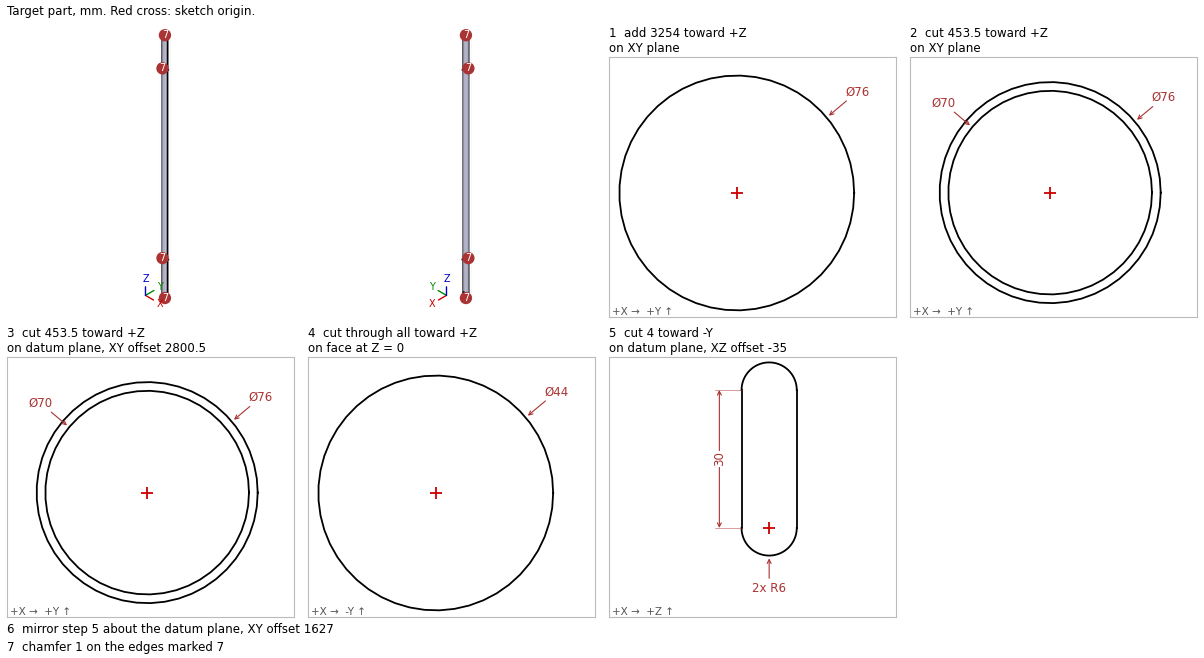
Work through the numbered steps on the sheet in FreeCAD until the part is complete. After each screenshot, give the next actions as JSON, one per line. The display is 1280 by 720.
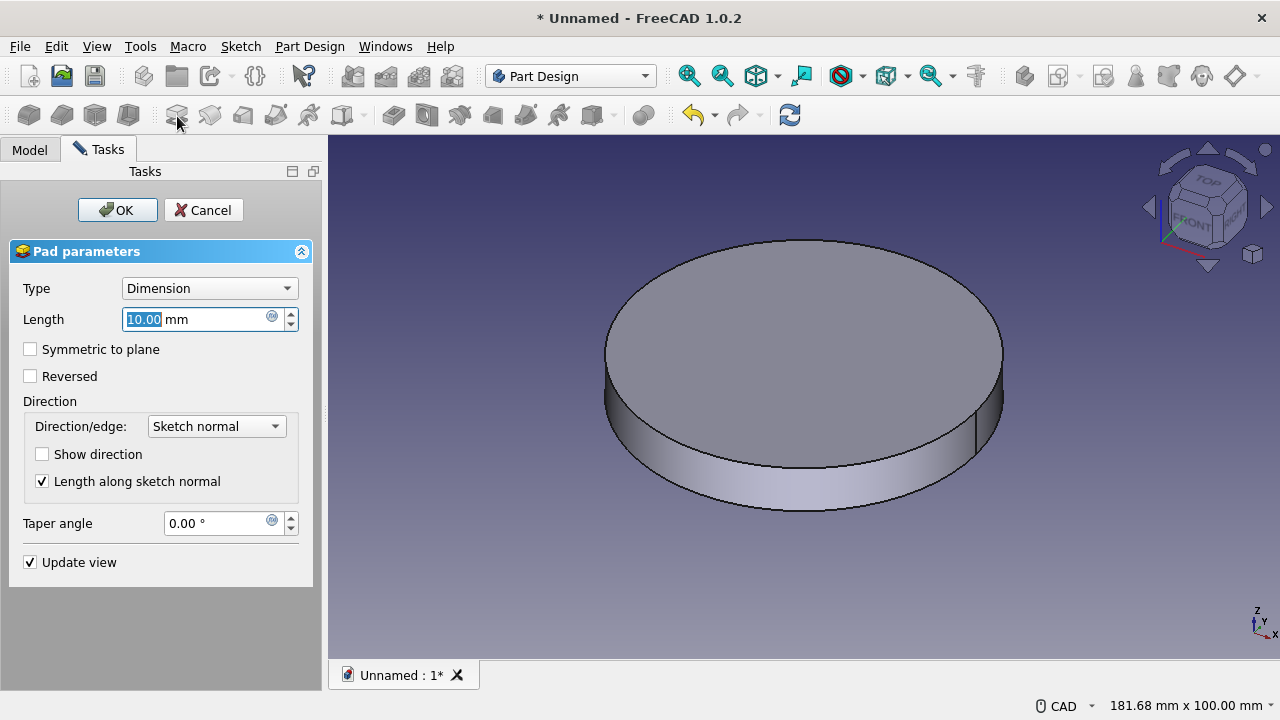
{"action": "type", "text": "3254"}
{"action": "key", "text": "Tab"}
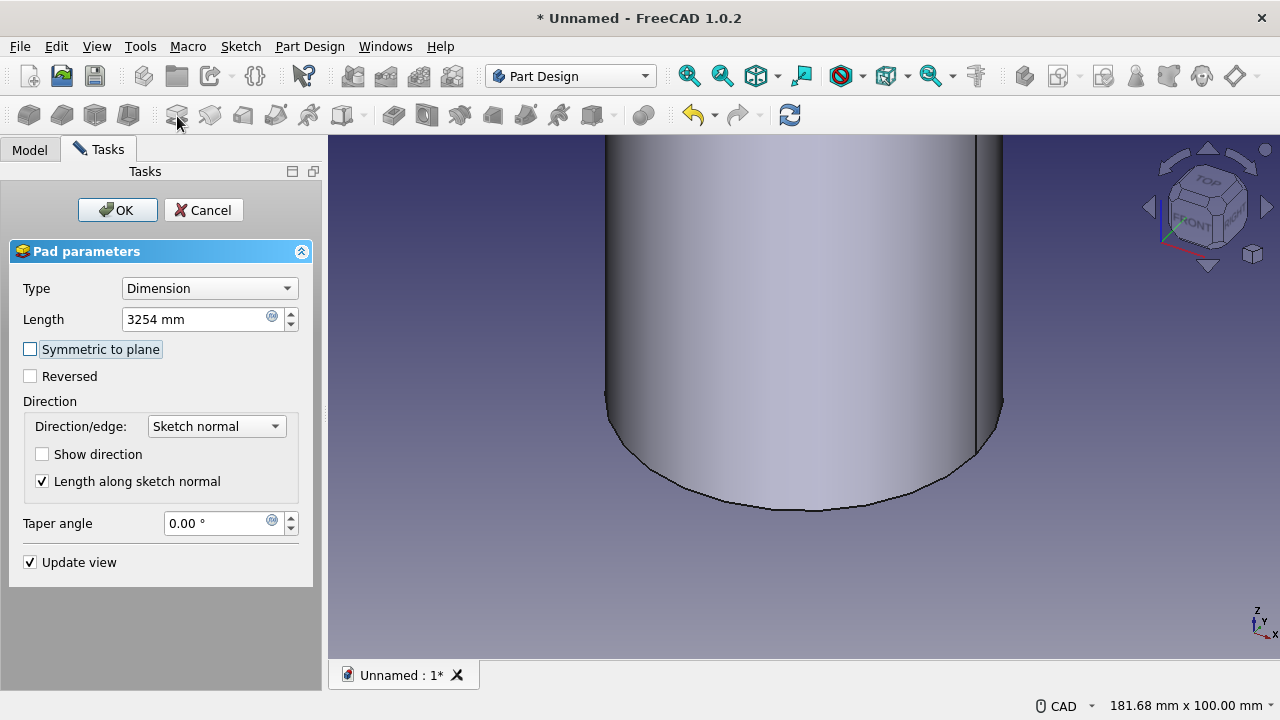
{"action": "left_click", "coordinate": [118, 210]}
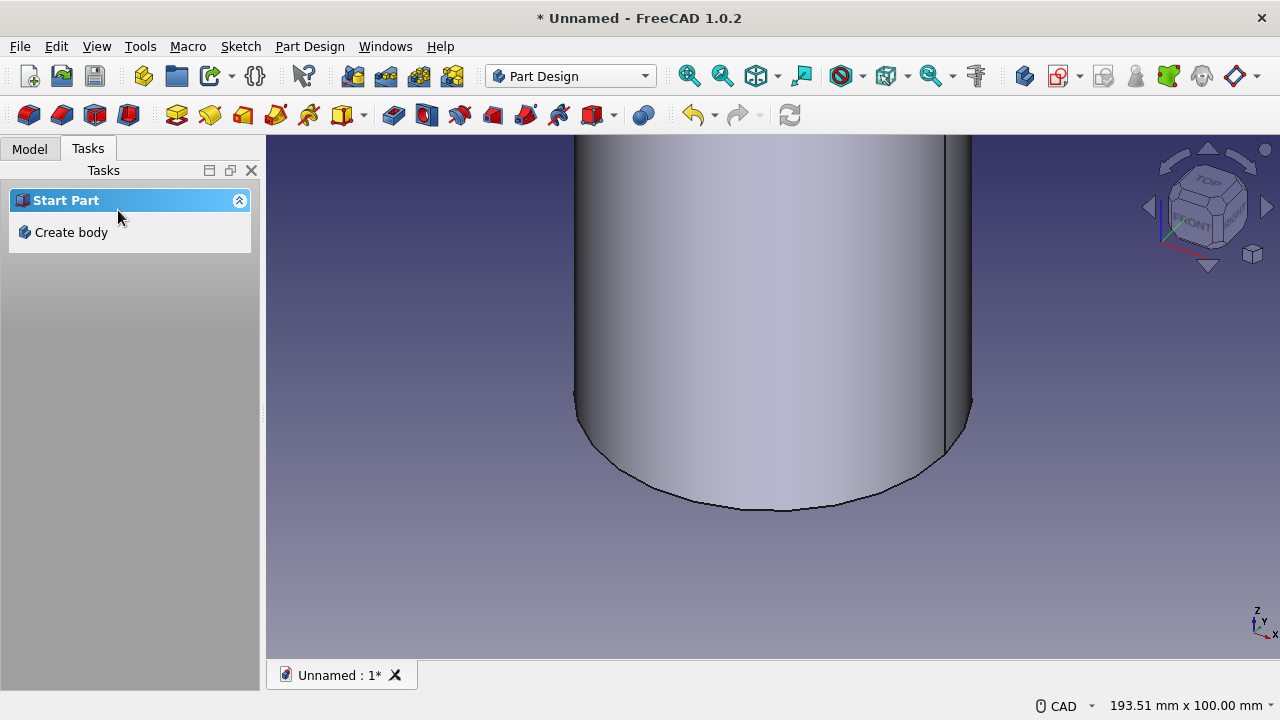
{"action": "left_click", "coordinate": [690, 76]}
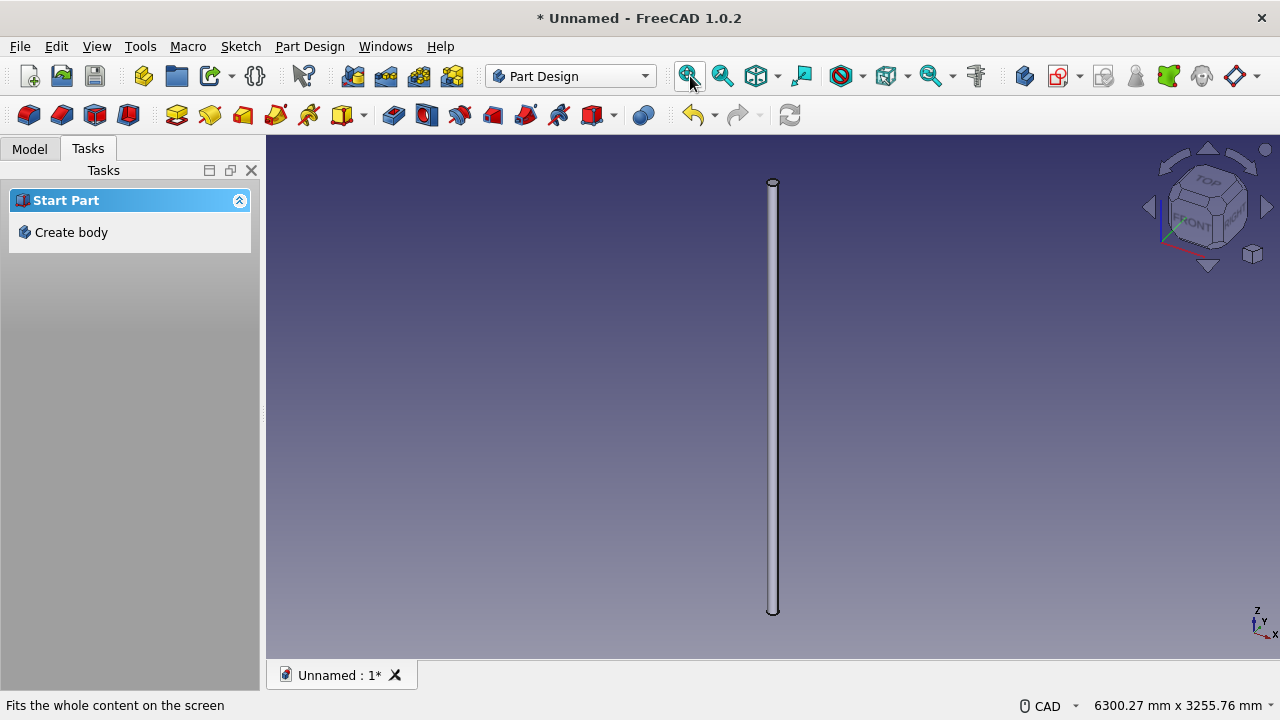
{"action": "left_click", "coordinate": [1058, 76]}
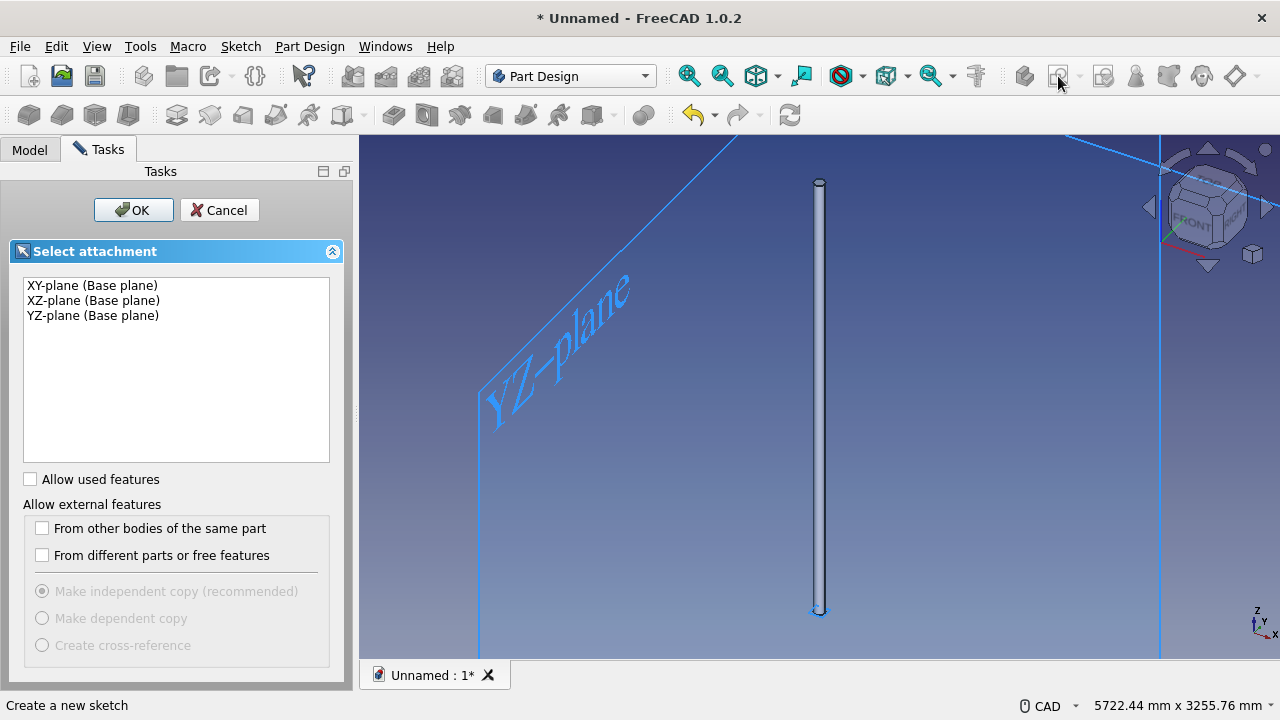
{"action": "left_click", "coordinate": [84, 286]}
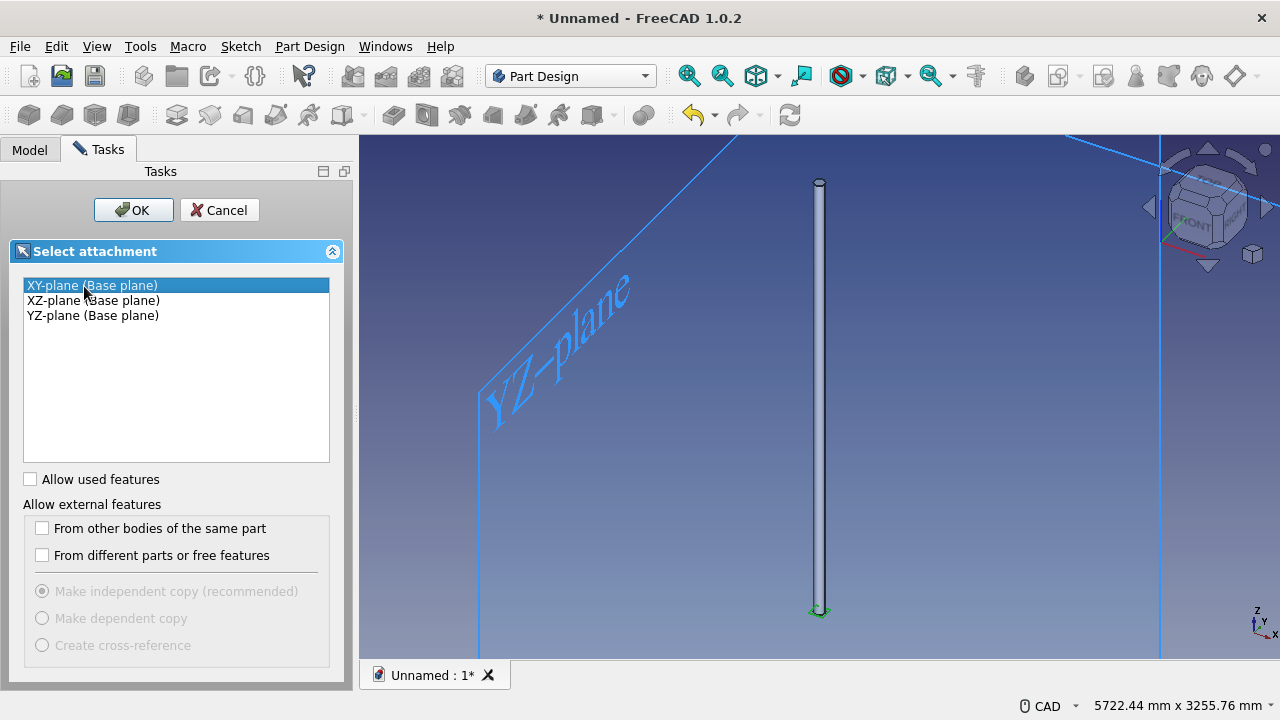
{"action": "left_click", "coordinate": [134, 210]}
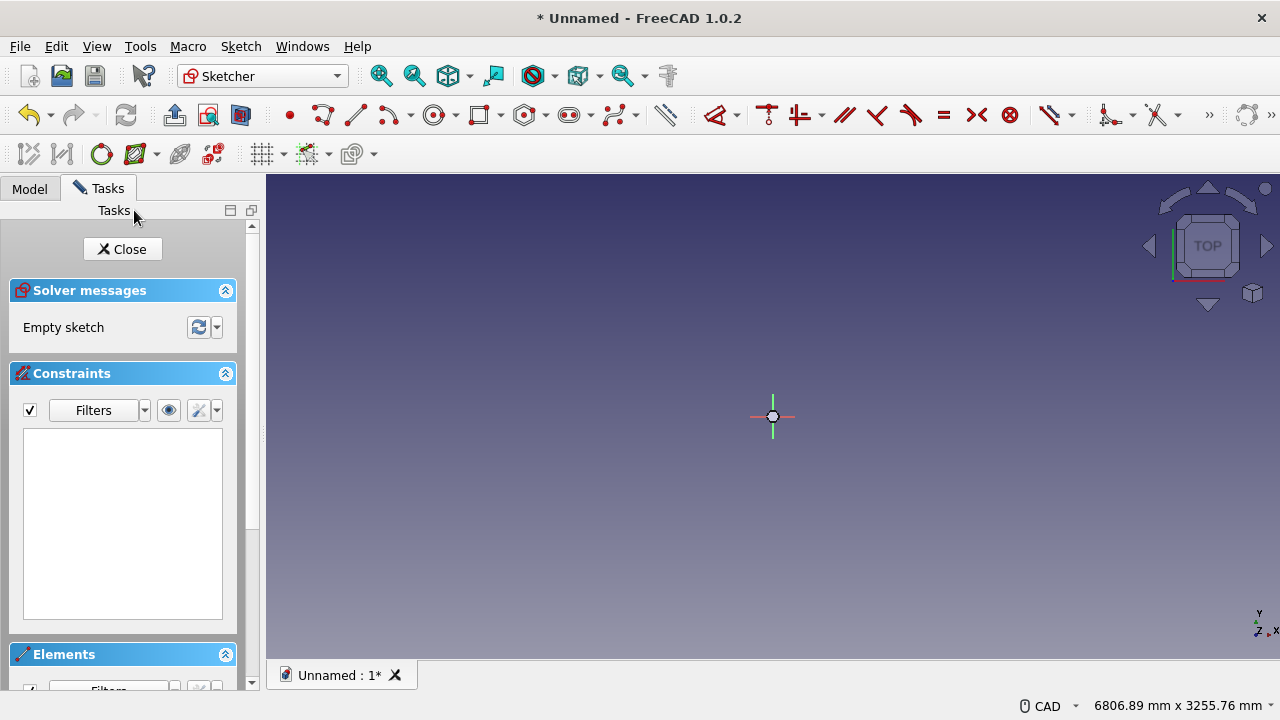
{"action": "left_click", "coordinate": [241, 116]}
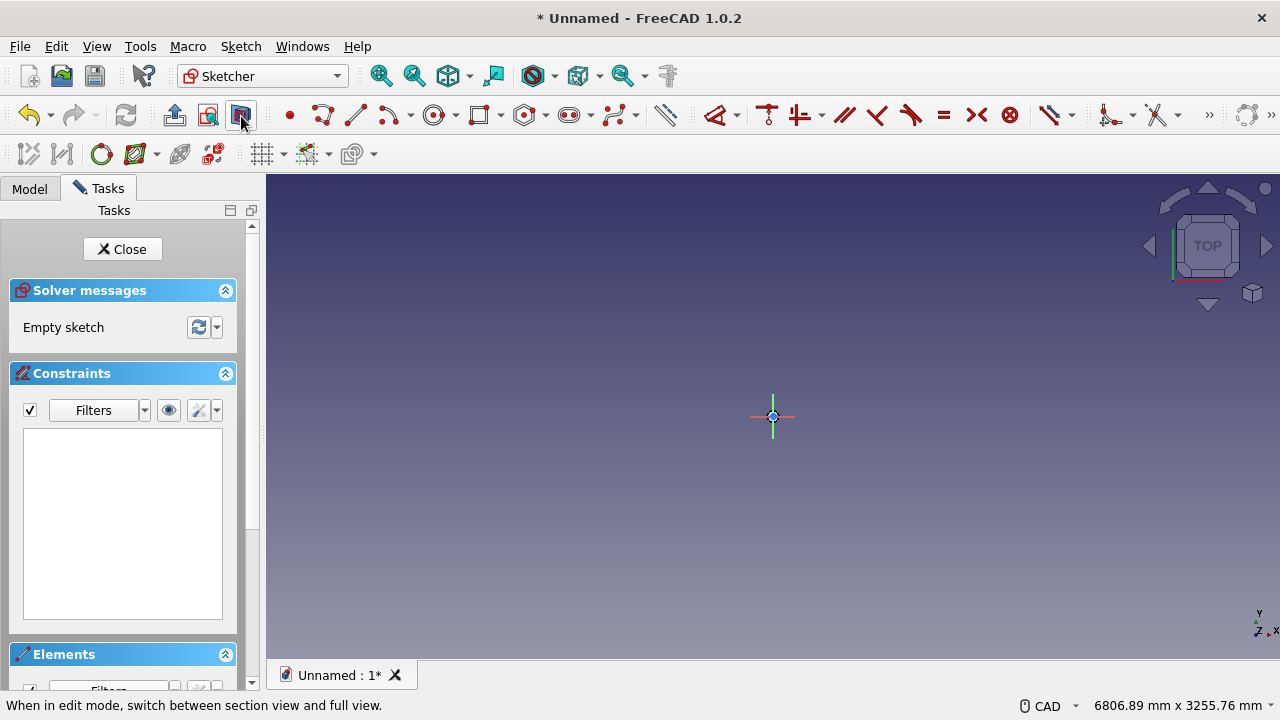
{"action": "scroll", "coordinate": [777, 416], "scroll_direction": "up", "scroll_amount": 15}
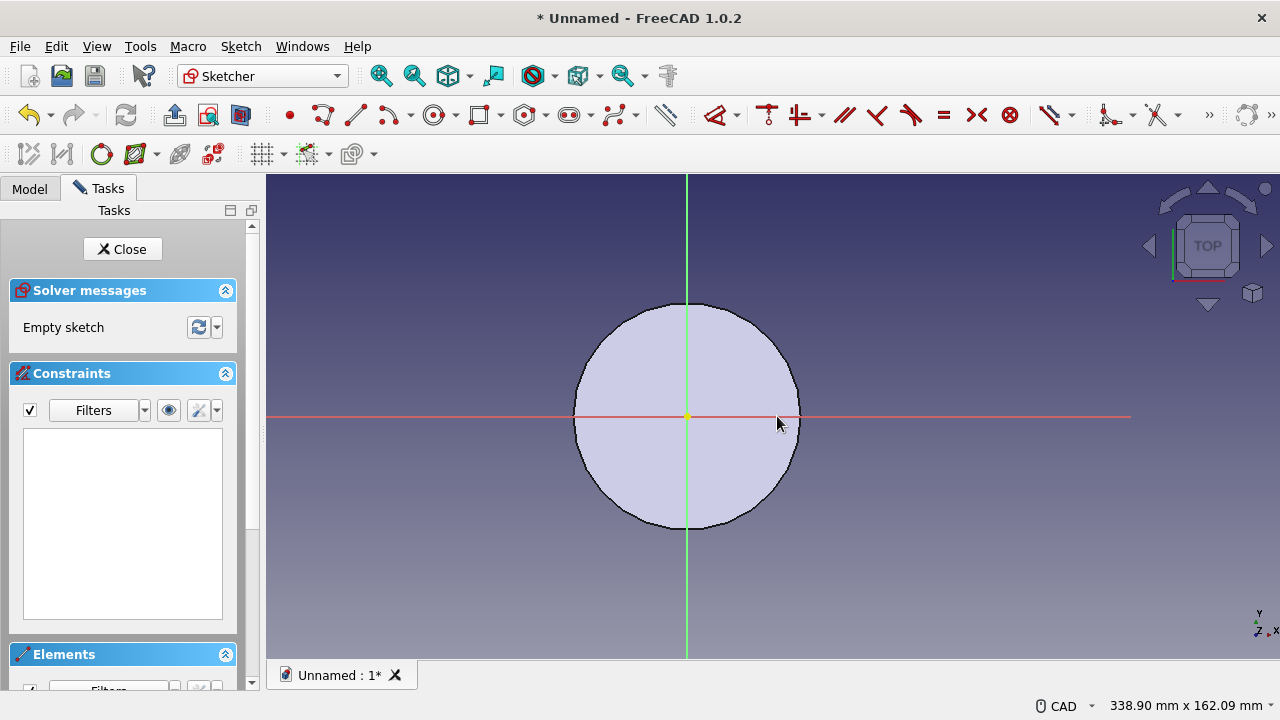
{"action": "left_click", "coordinate": [434, 116]}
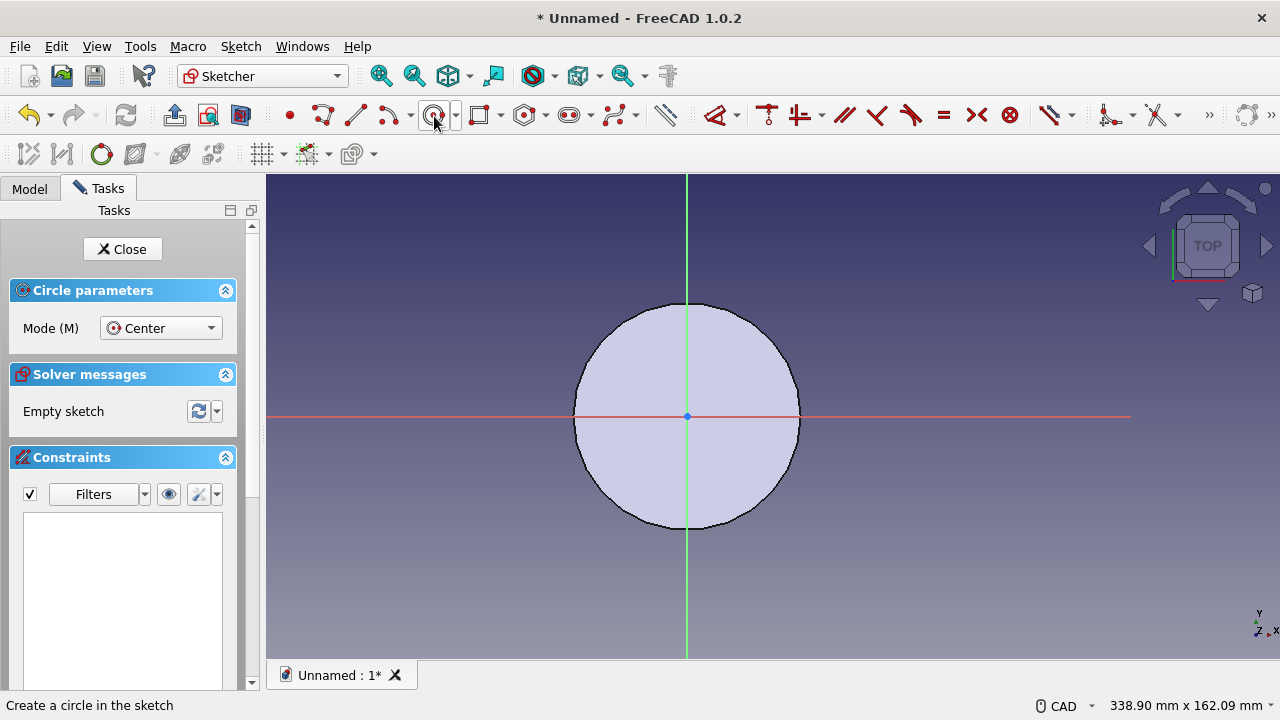
{"action": "left_click", "coordinate": [687, 416]}
{"action": "left_click", "coordinate": [767, 336]}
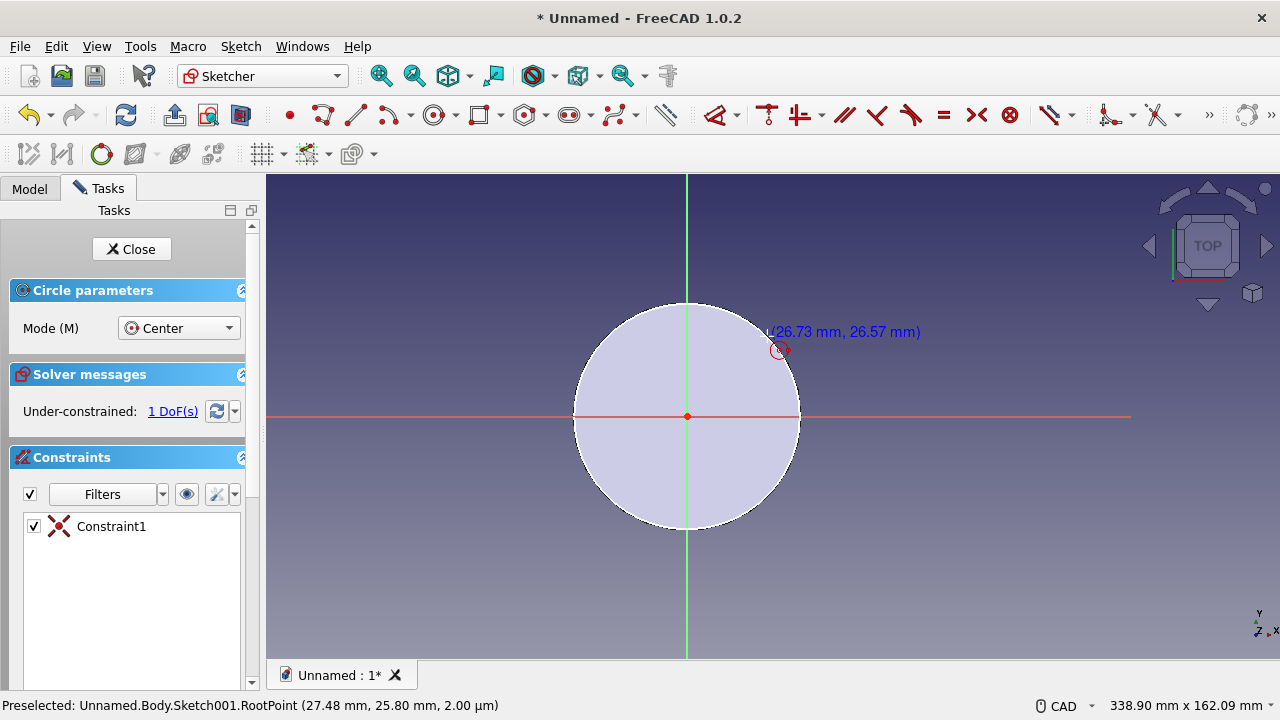
{"action": "left_click", "coordinate": [687, 416]}